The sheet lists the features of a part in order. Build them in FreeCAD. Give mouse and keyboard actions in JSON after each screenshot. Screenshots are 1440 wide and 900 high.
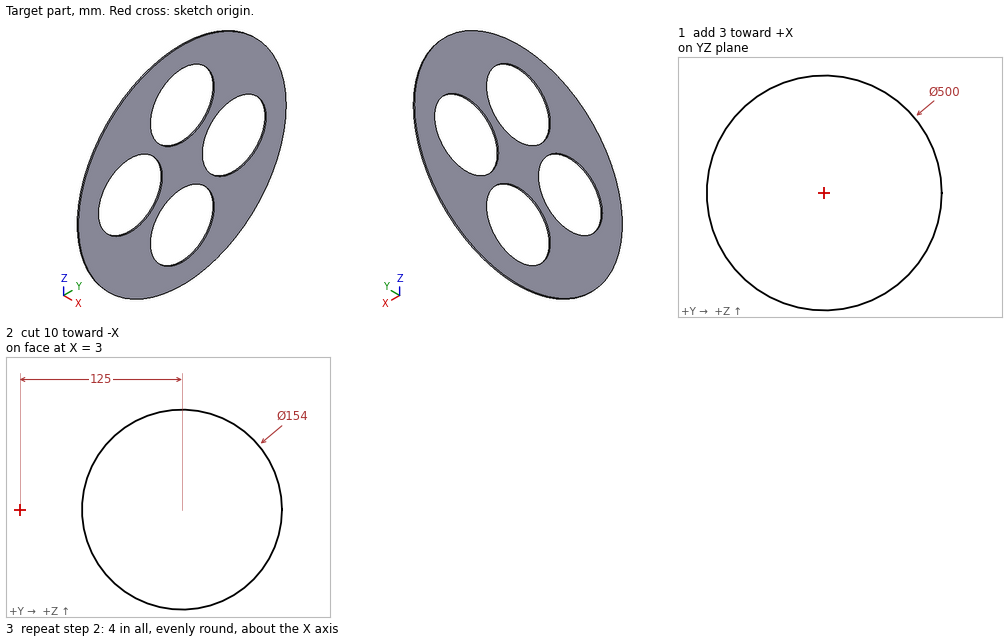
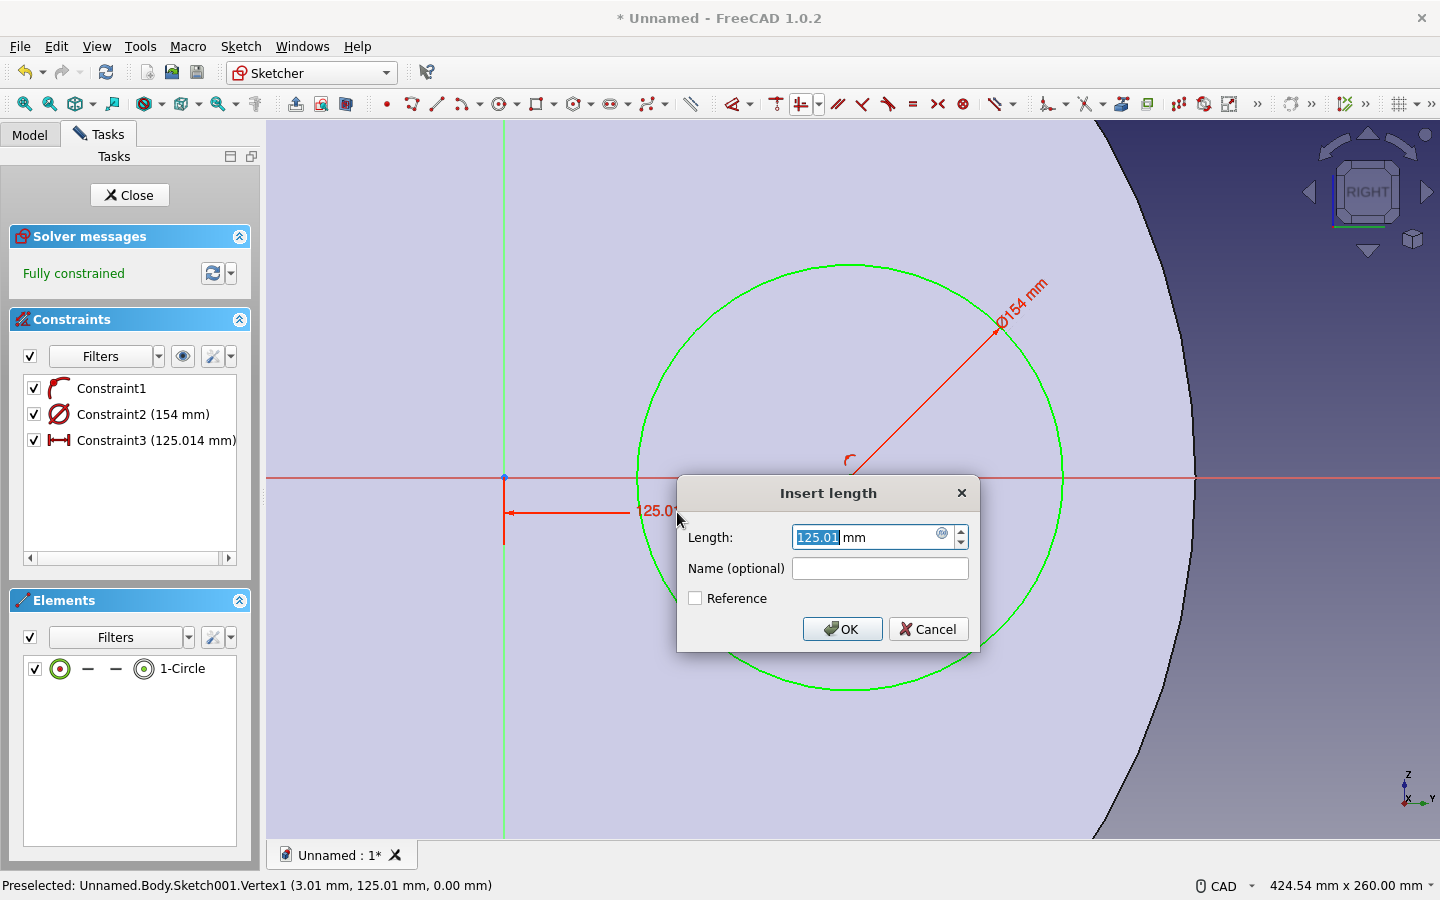
{"action": "type", "text": "125"}
{"action": "key", "text": "Return"}
{"action": "key", "text": "Escape"}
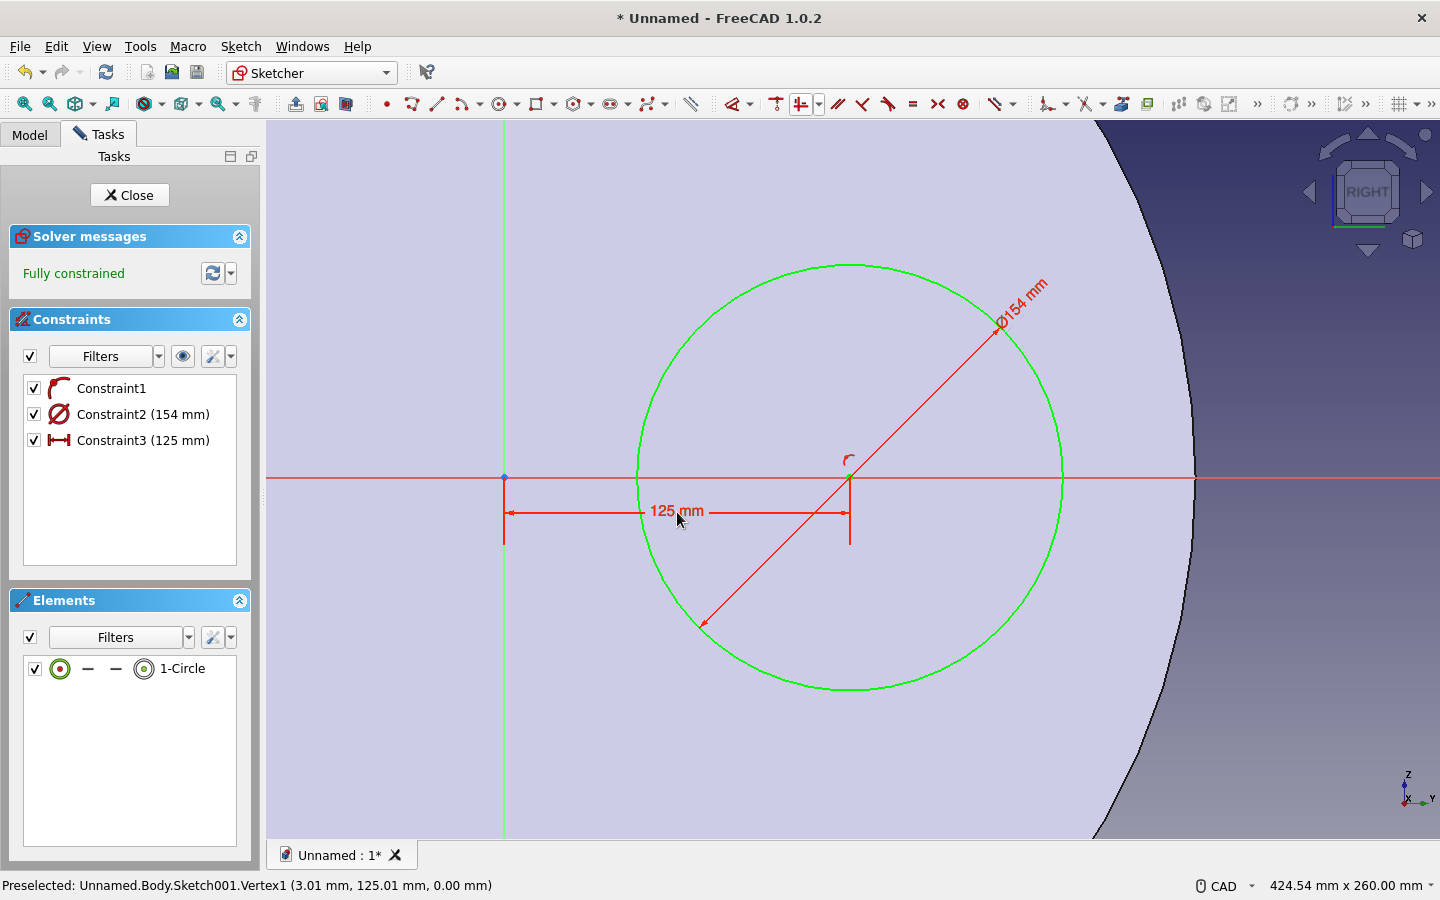
{"action": "left_click", "coordinate": [130, 195]}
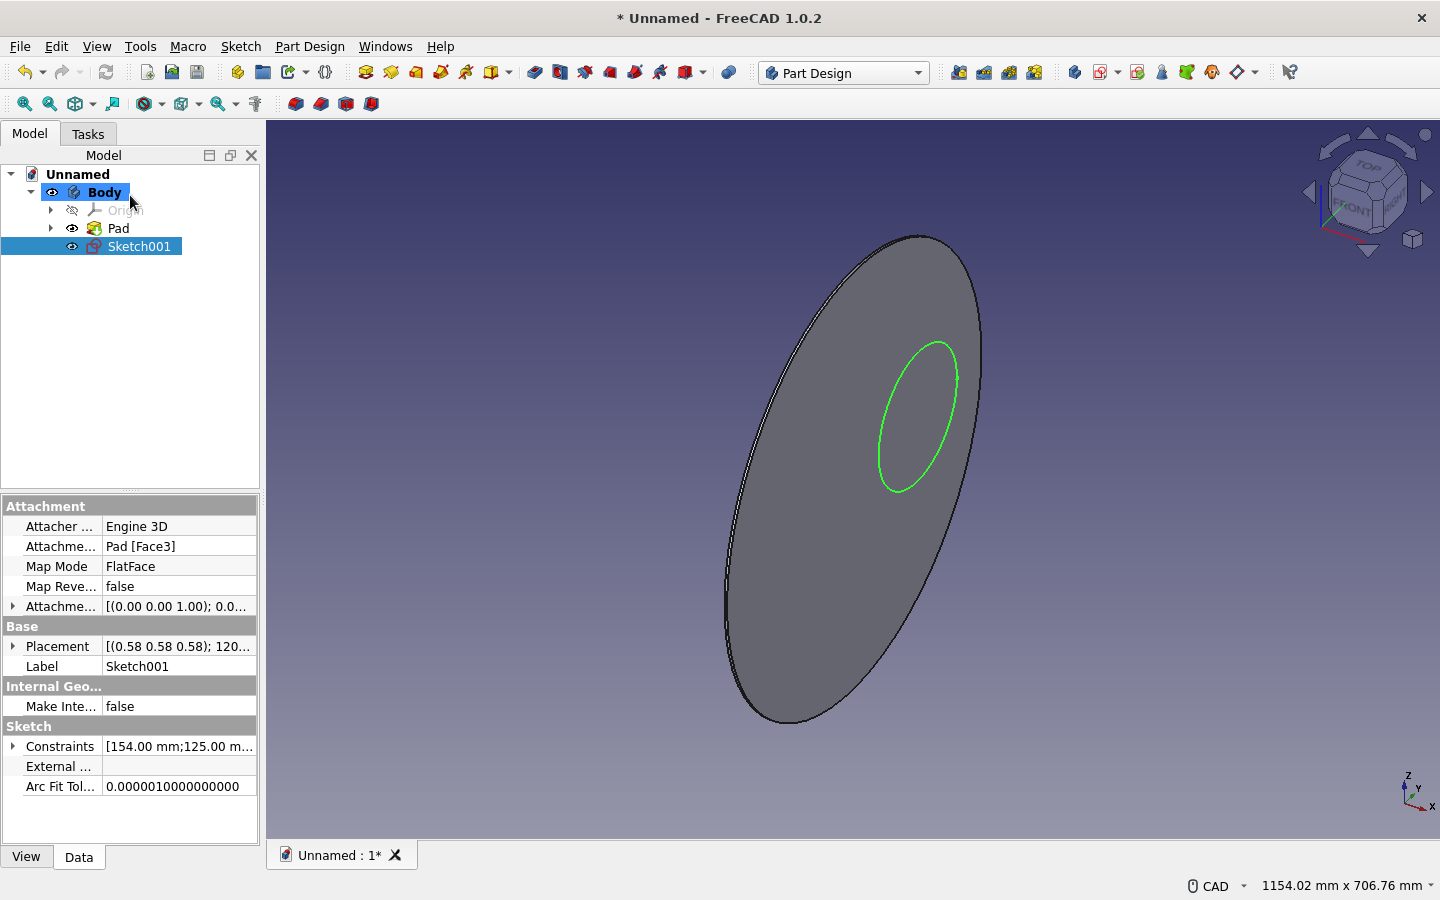
{"action": "left_click", "coordinate": [535, 72]}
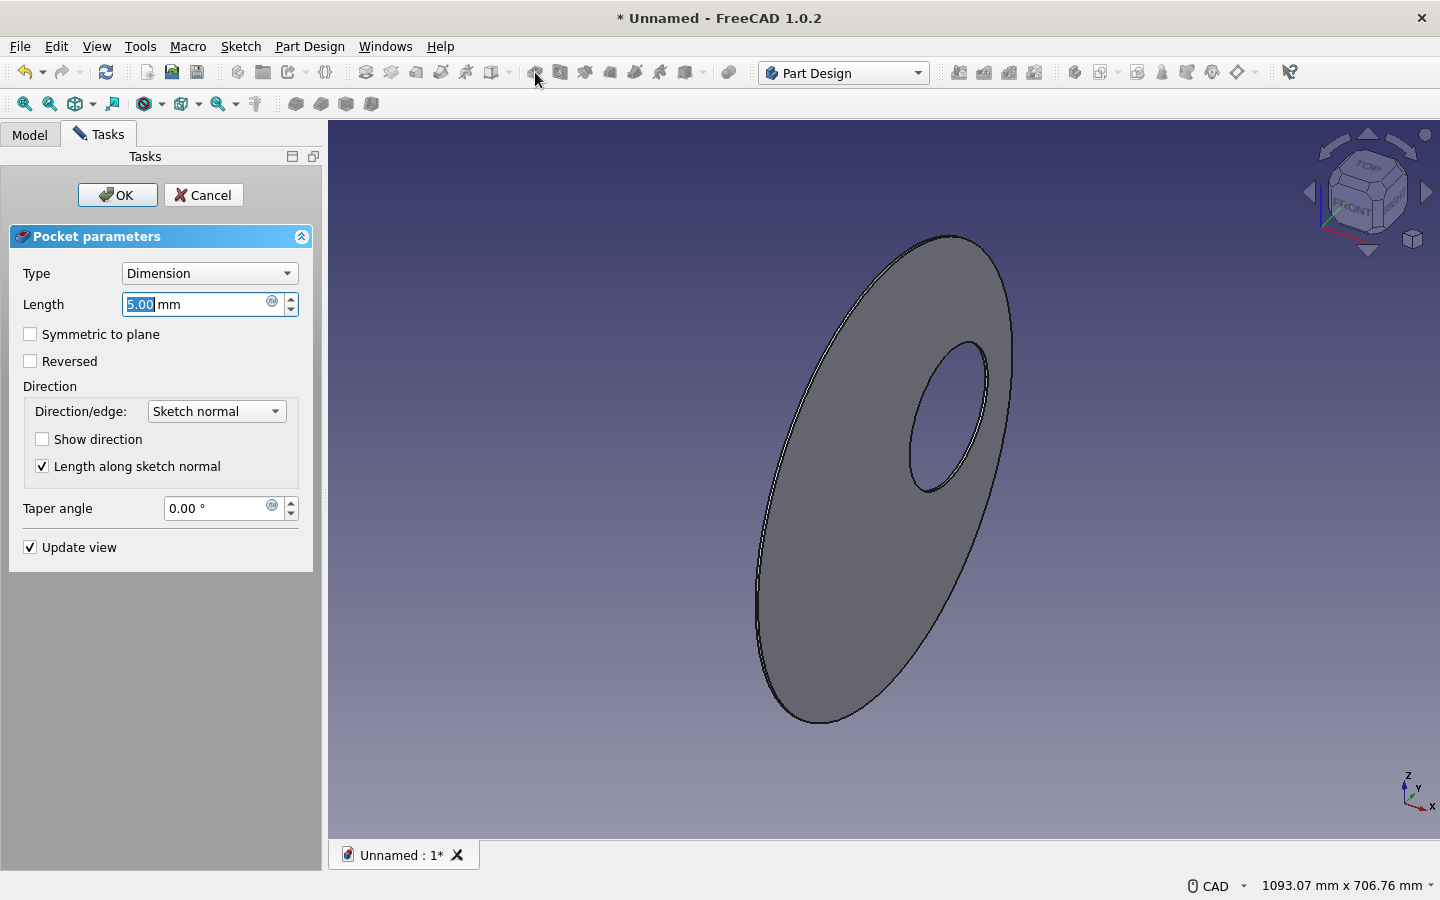
{"action": "type", "text": "10"}
{"action": "key", "text": "Tab"}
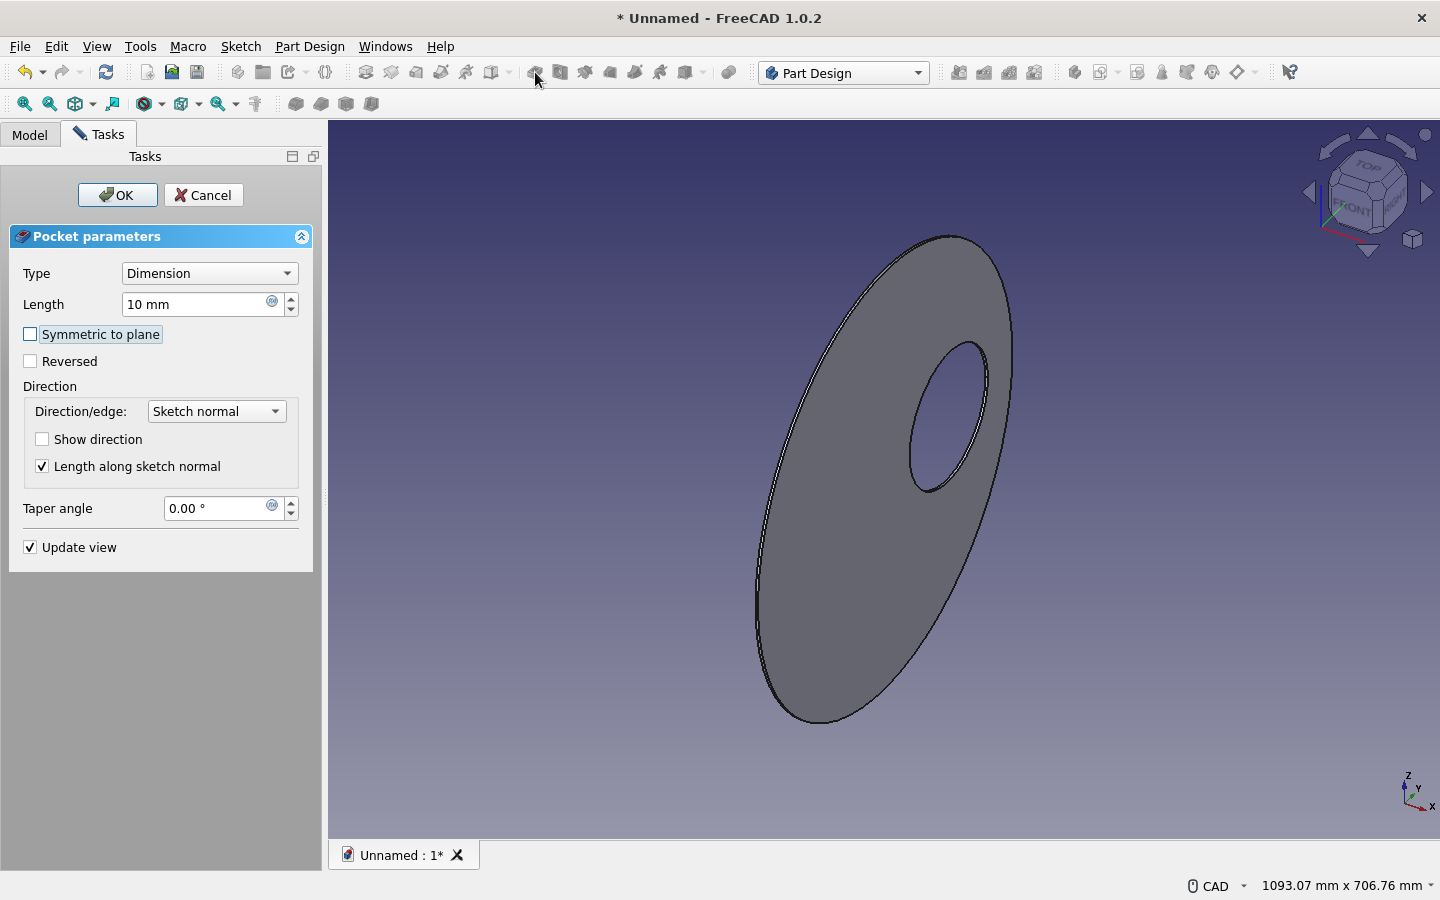
{"action": "left_click", "coordinate": [118, 195]}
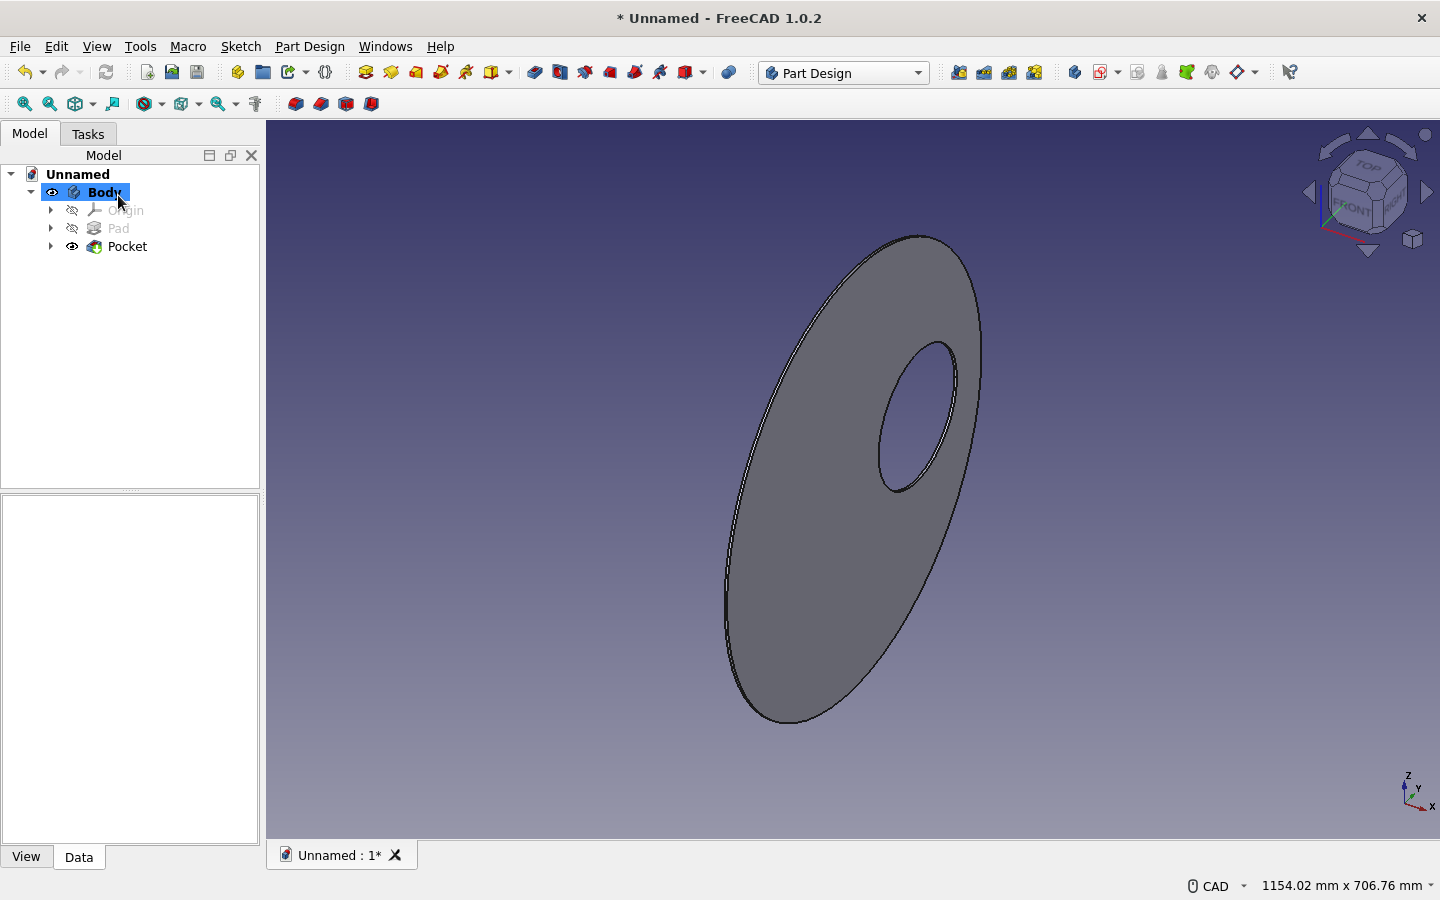
{"action": "left_click", "coordinate": [117, 246]}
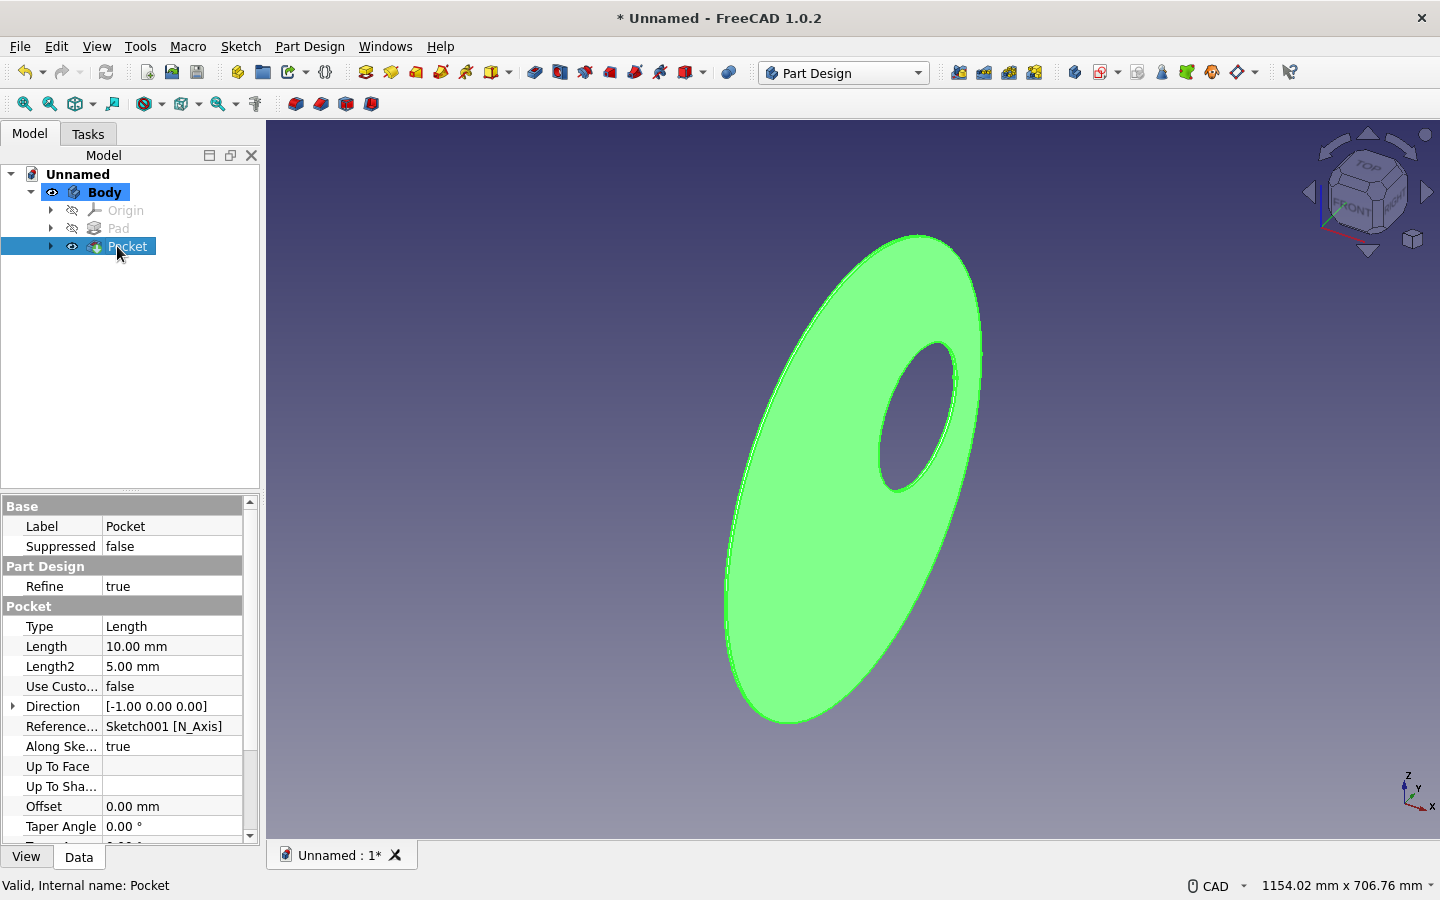
{"action": "left_click", "coordinate": [1009, 72]}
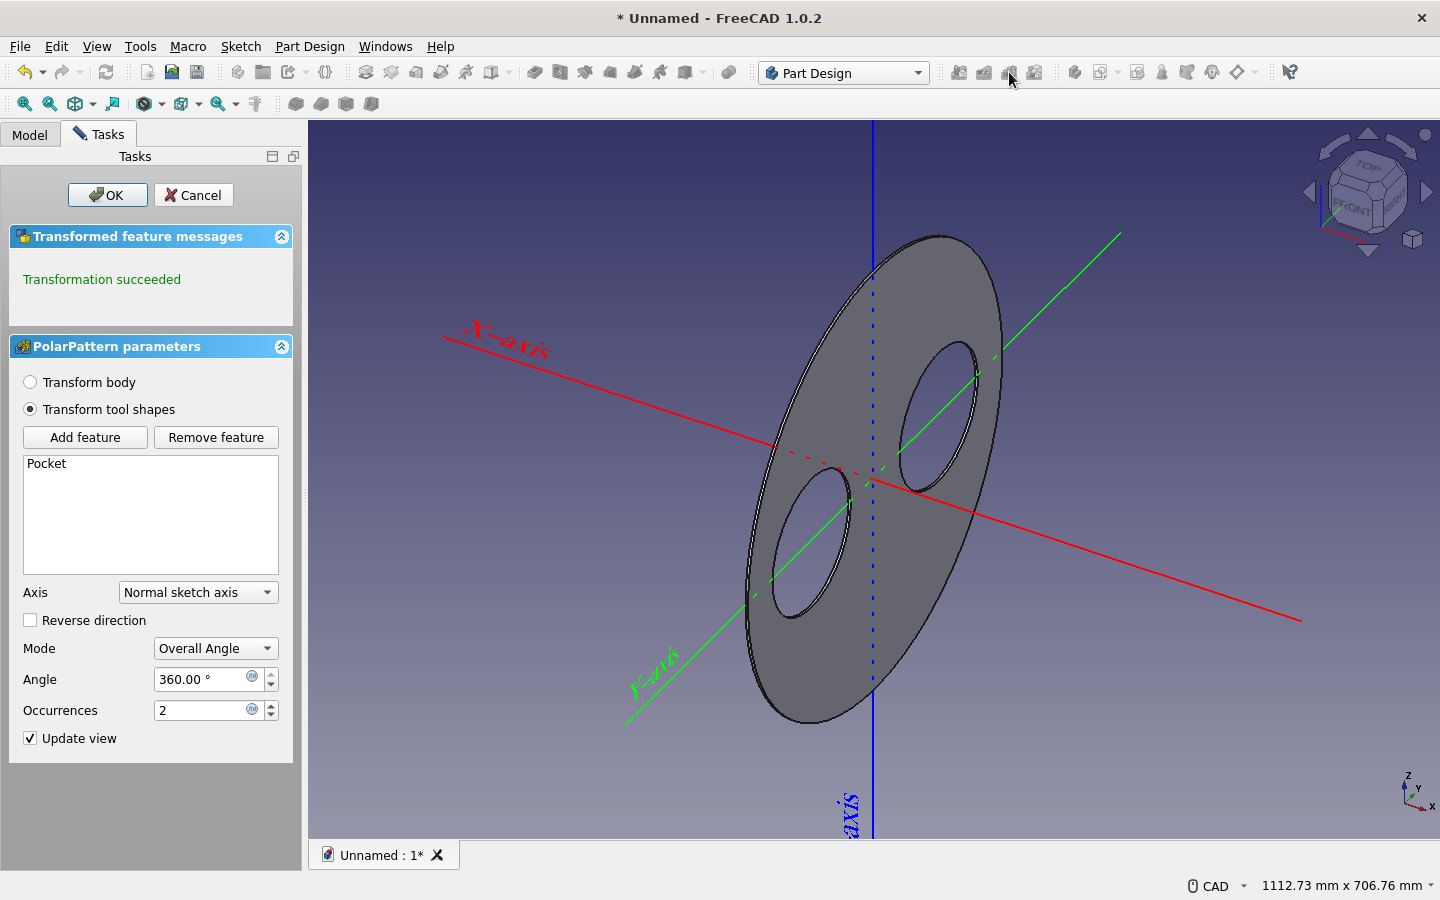
{"action": "left_click", "coordinate": [199, 592]}